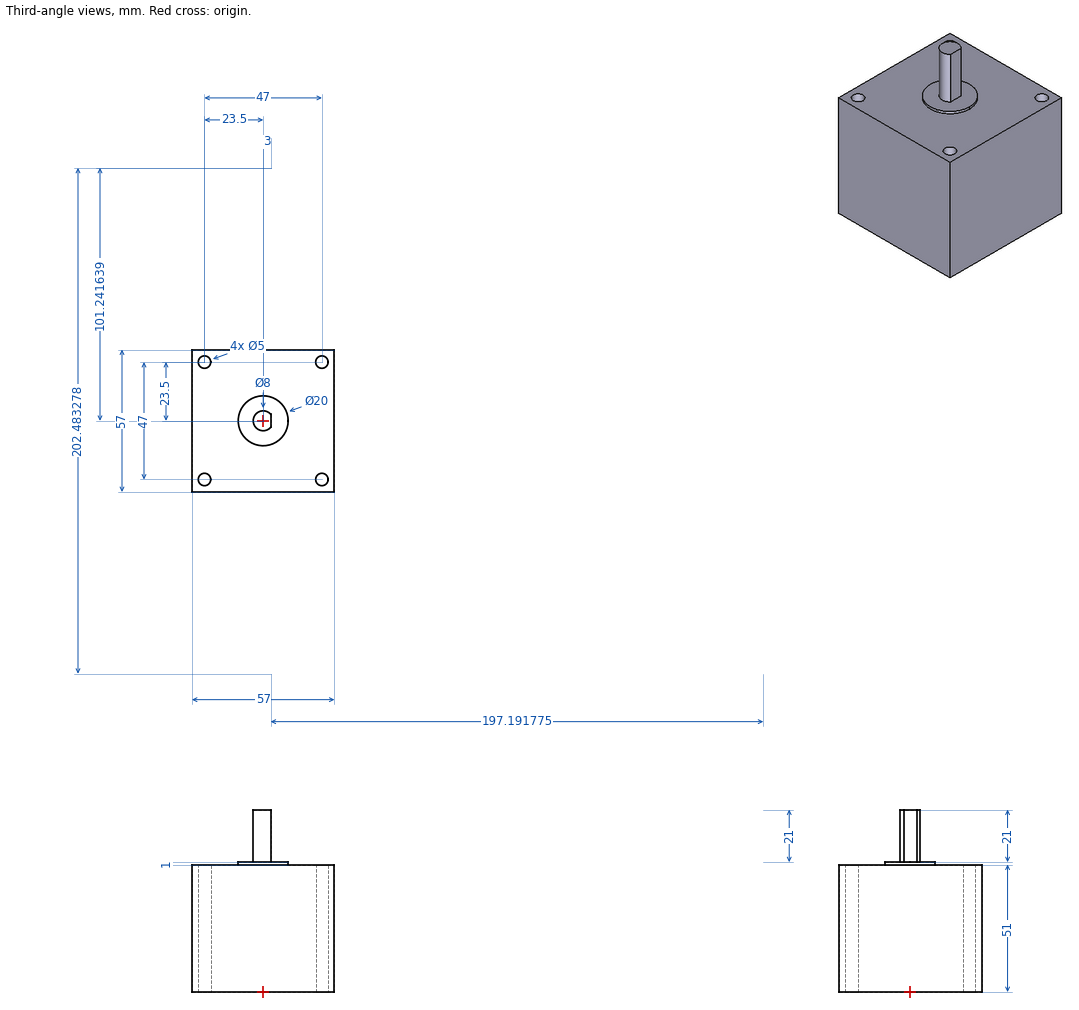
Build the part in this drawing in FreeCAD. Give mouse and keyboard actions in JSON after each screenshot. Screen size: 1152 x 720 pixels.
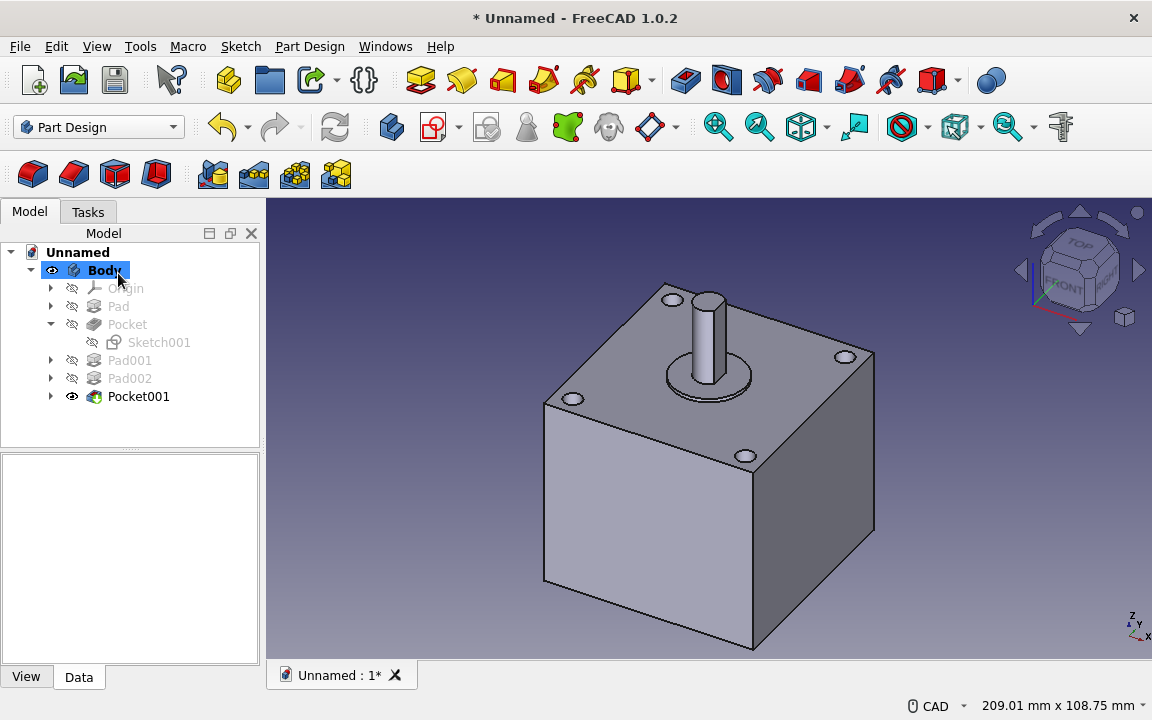
{"action": "key", "text": "0"}